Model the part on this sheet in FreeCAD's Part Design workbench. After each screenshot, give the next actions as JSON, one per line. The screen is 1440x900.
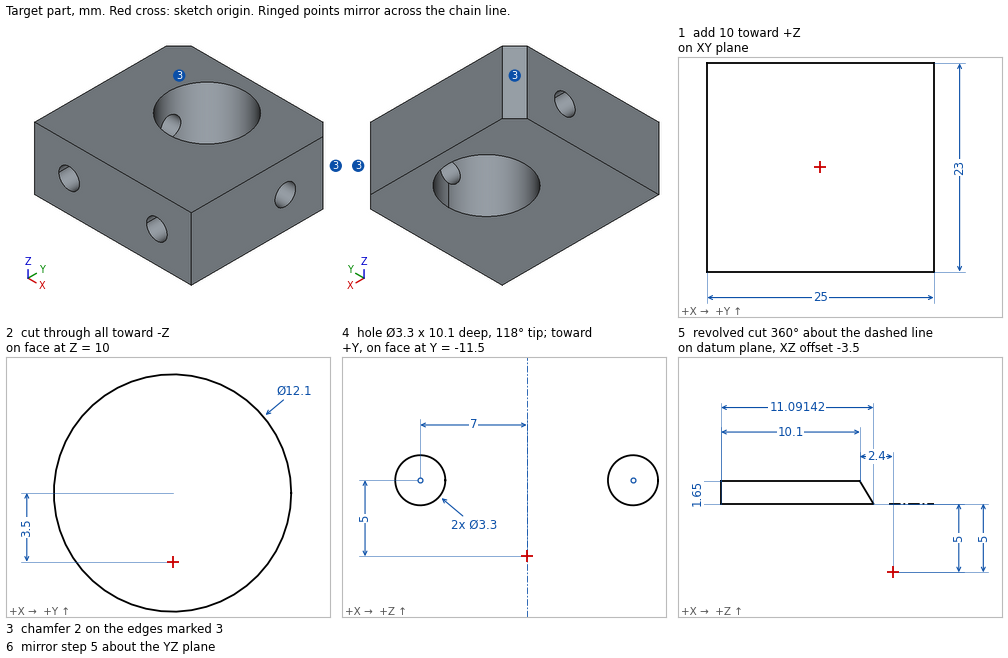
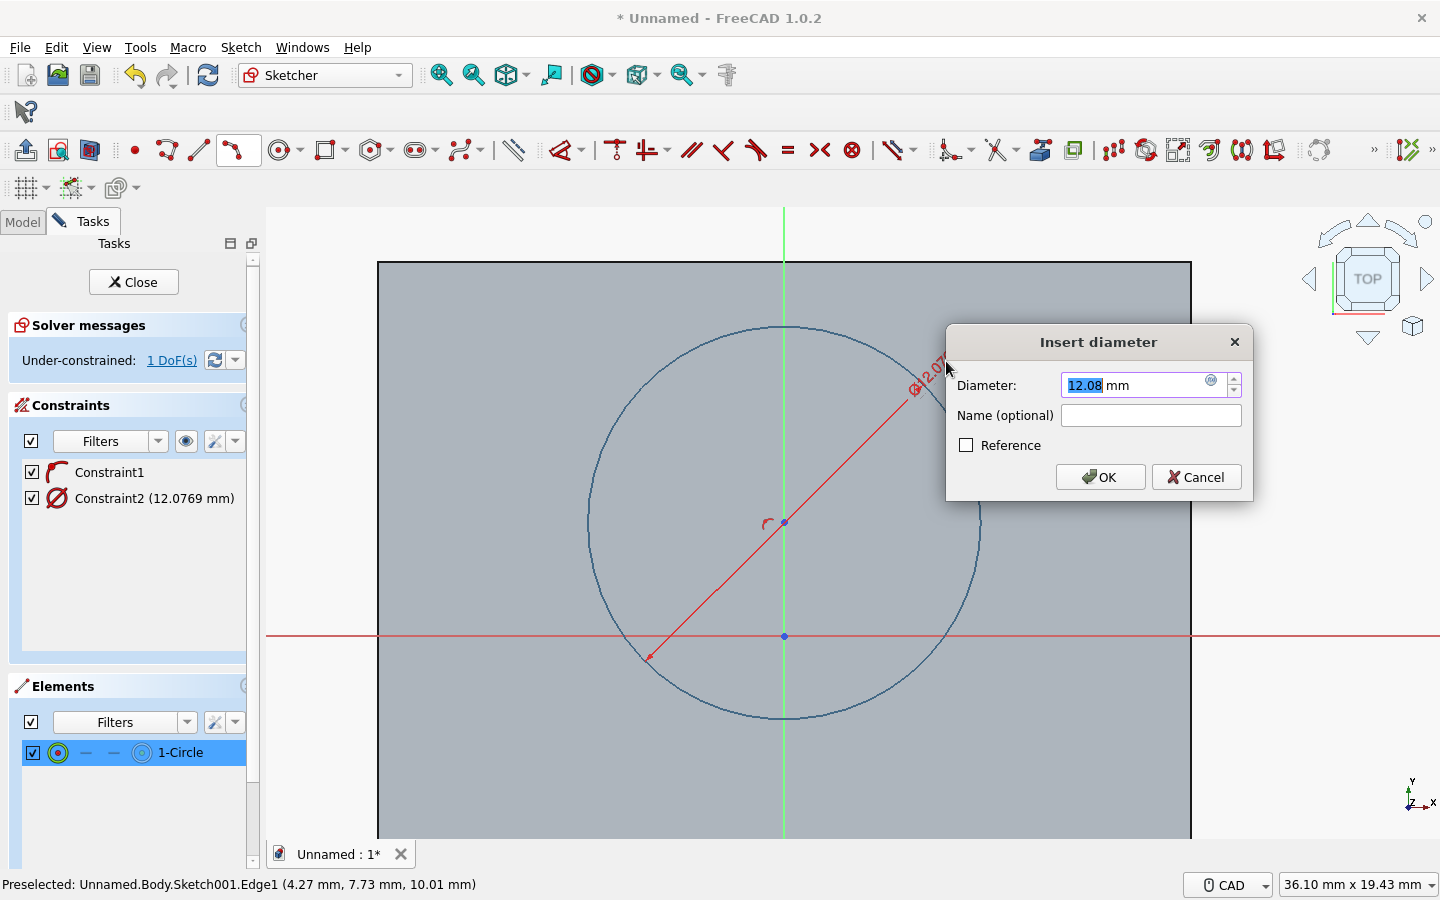
{"action": "type", "text": "12.1"}
{"action": "key", "text": "Return"}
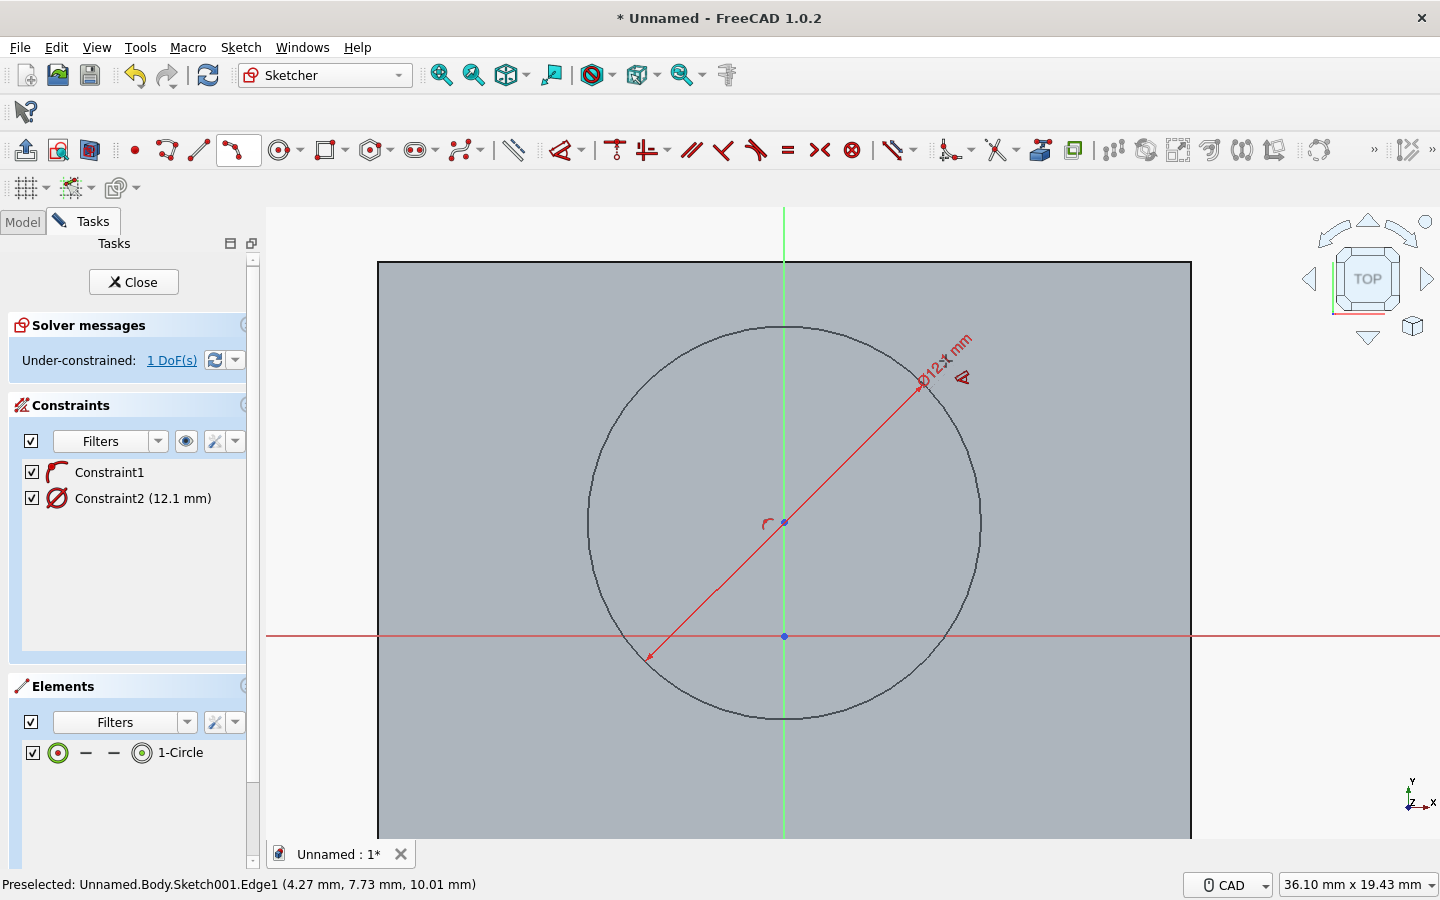
{"action": "left_click", "coordinate": [784, 523]}
{"action": "left_click", "coordinate": [818, 580]}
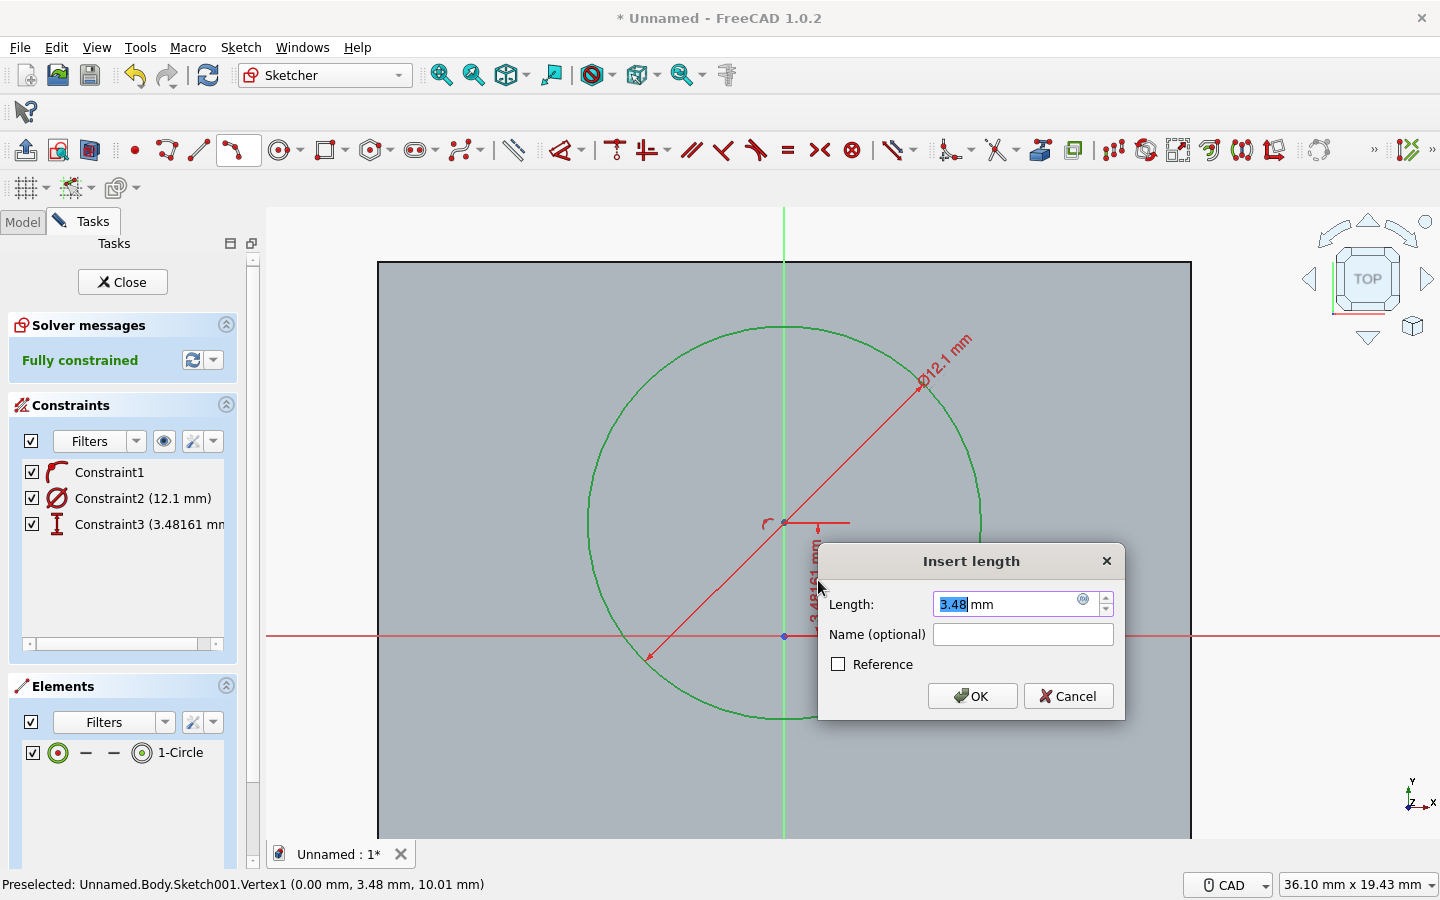
{"action": "type", "text": "3.5"}
{"action": "key", "text": "Return"}
{"action": "key", "text": "Escape"}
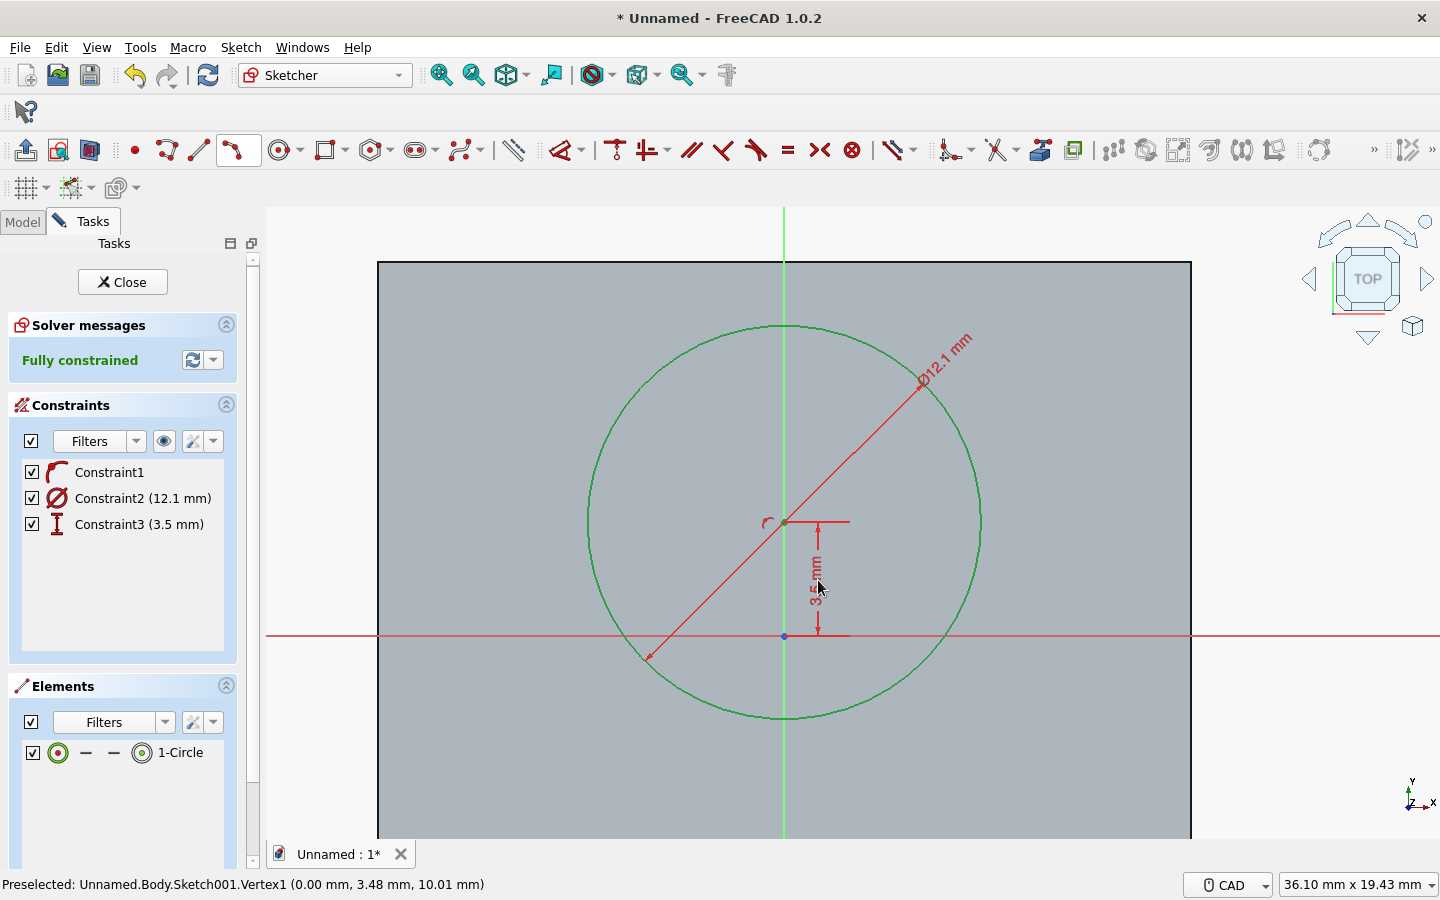
{"action": "left_click", "coordinate": [123, 282]}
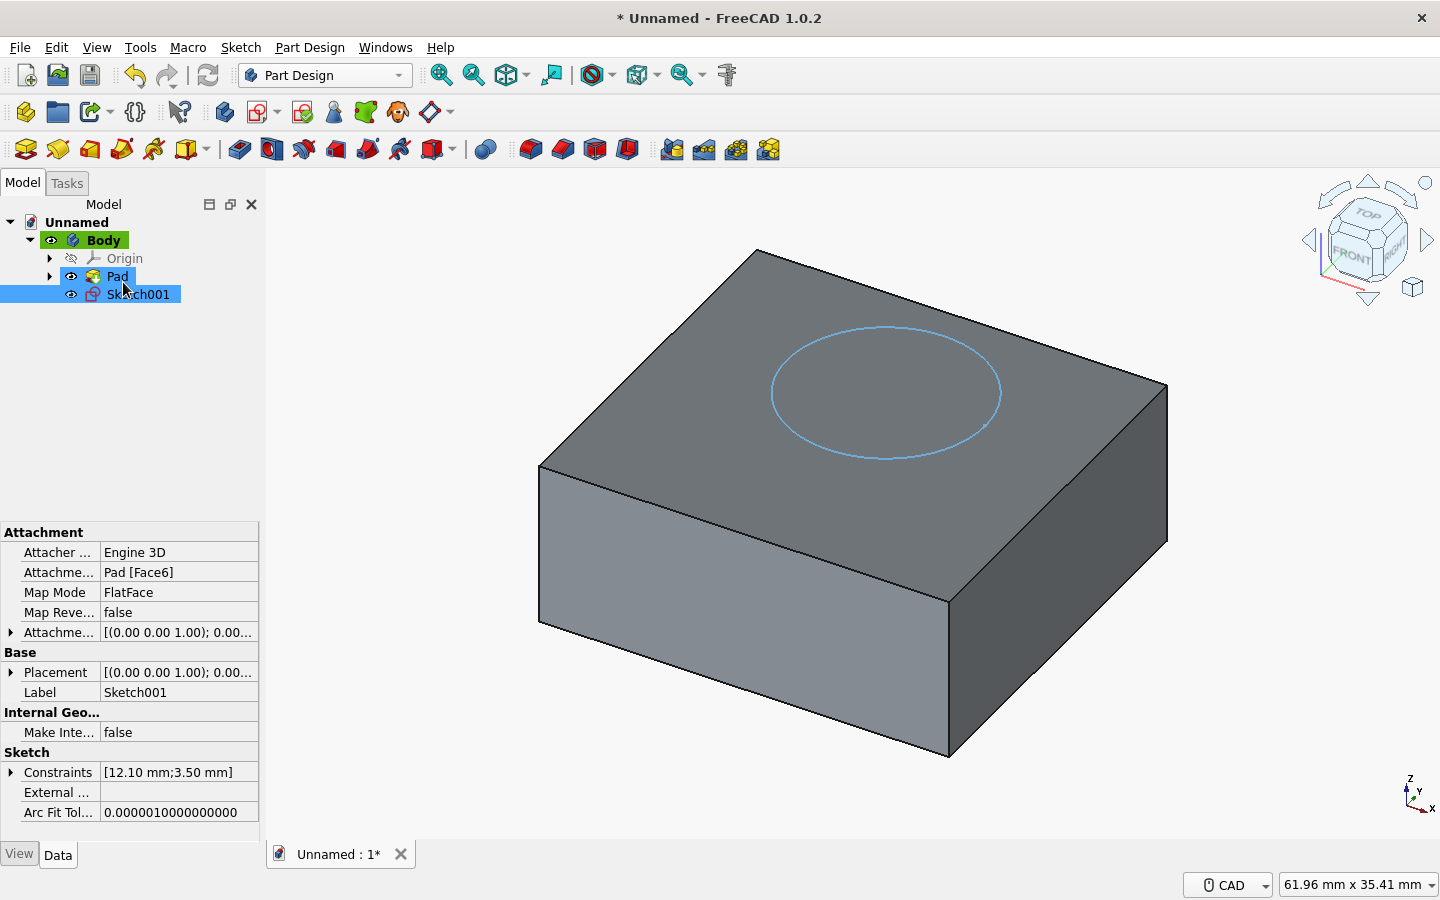
{"action": "left_click", "coordinate": [240, 150]}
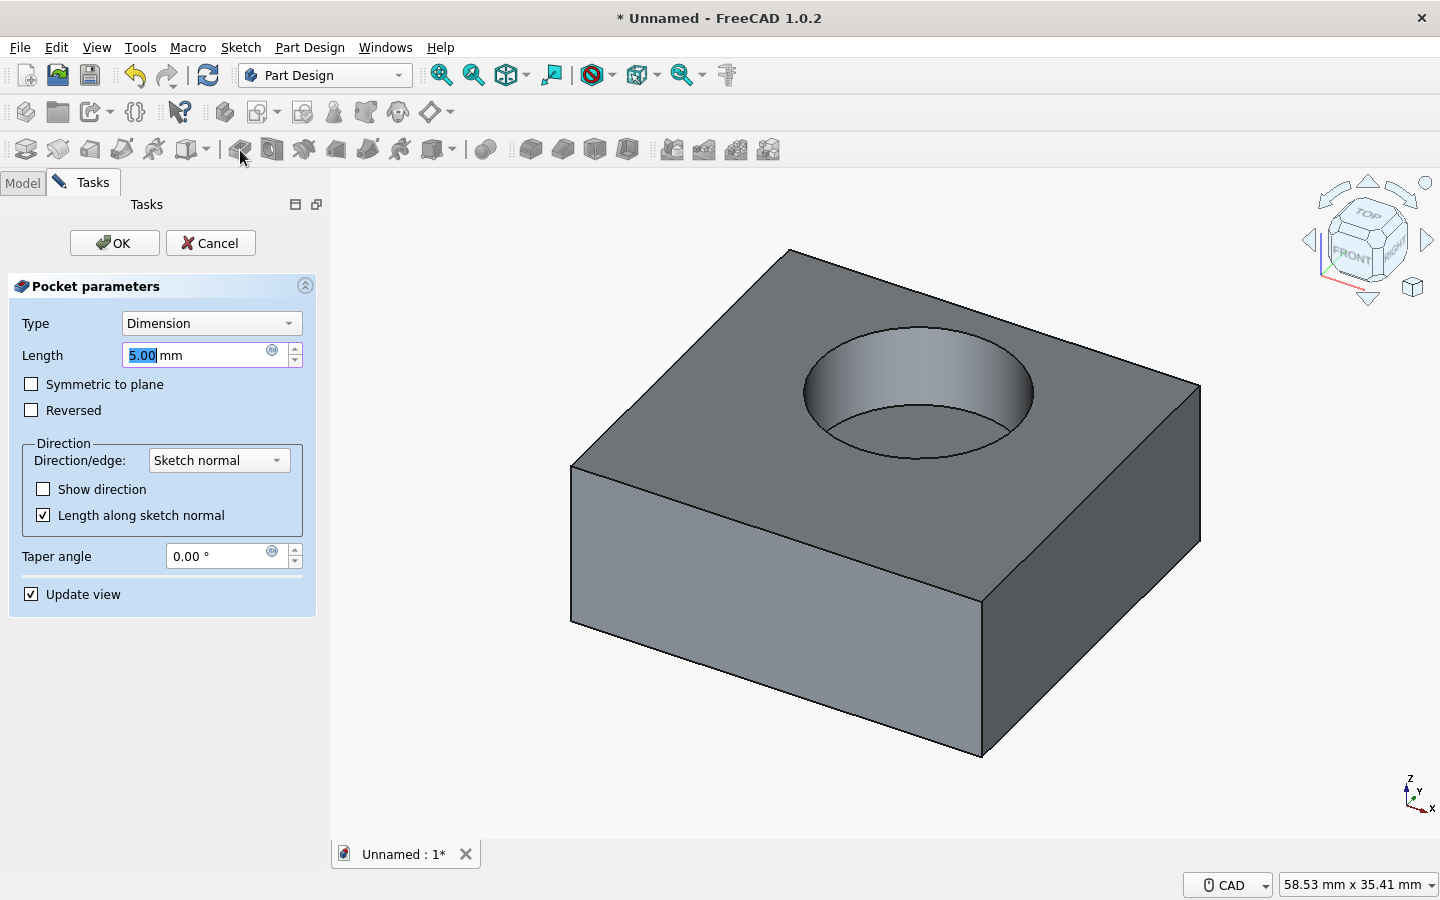
{"action": "left_click", "coordinate": [212, 324]}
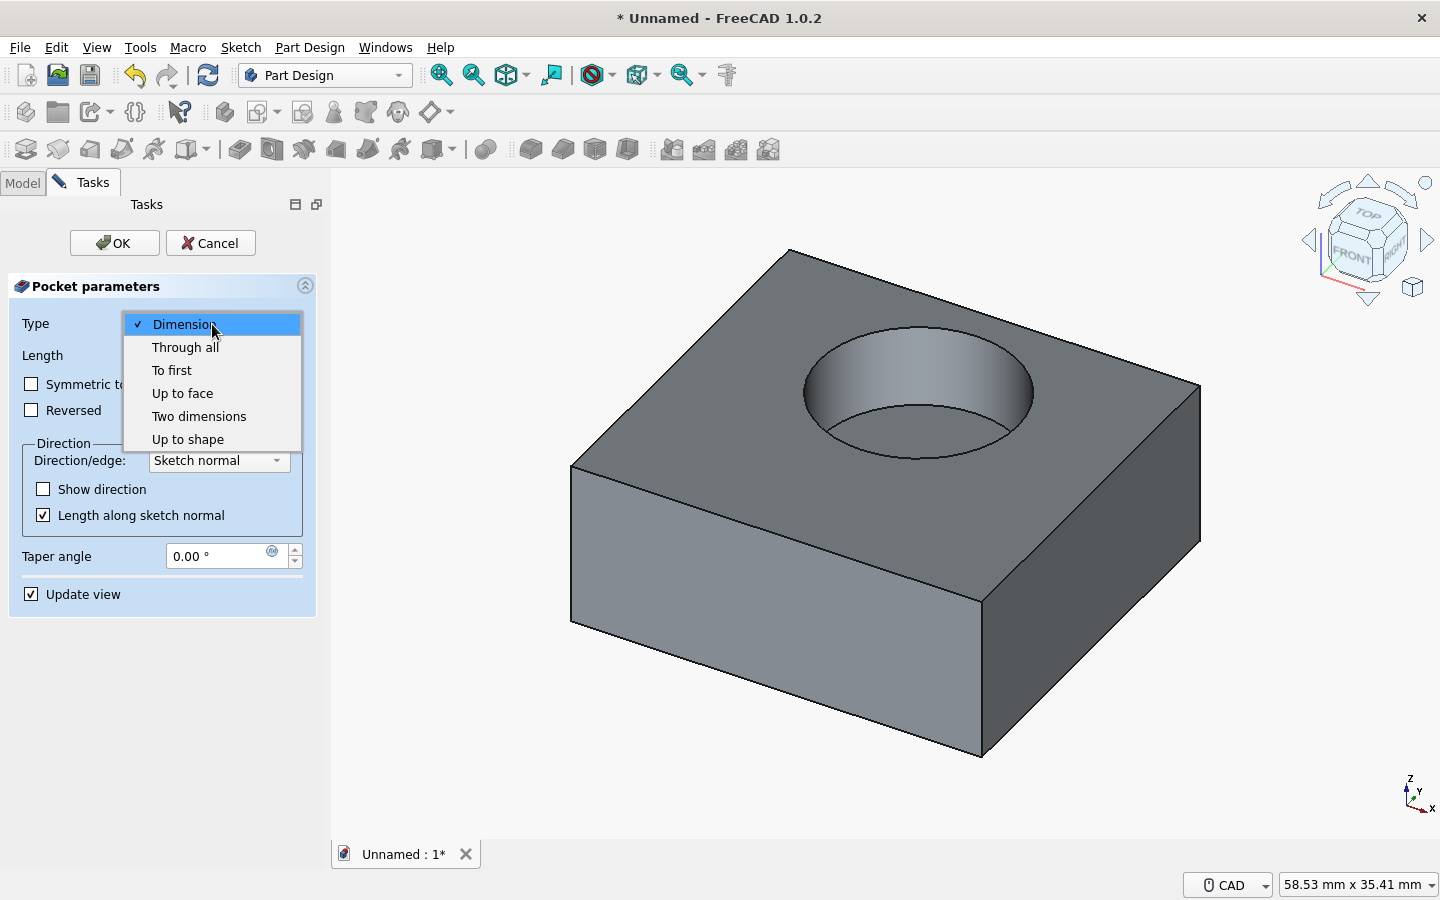
{"action": "left_click", "coordinate": [212, 348]}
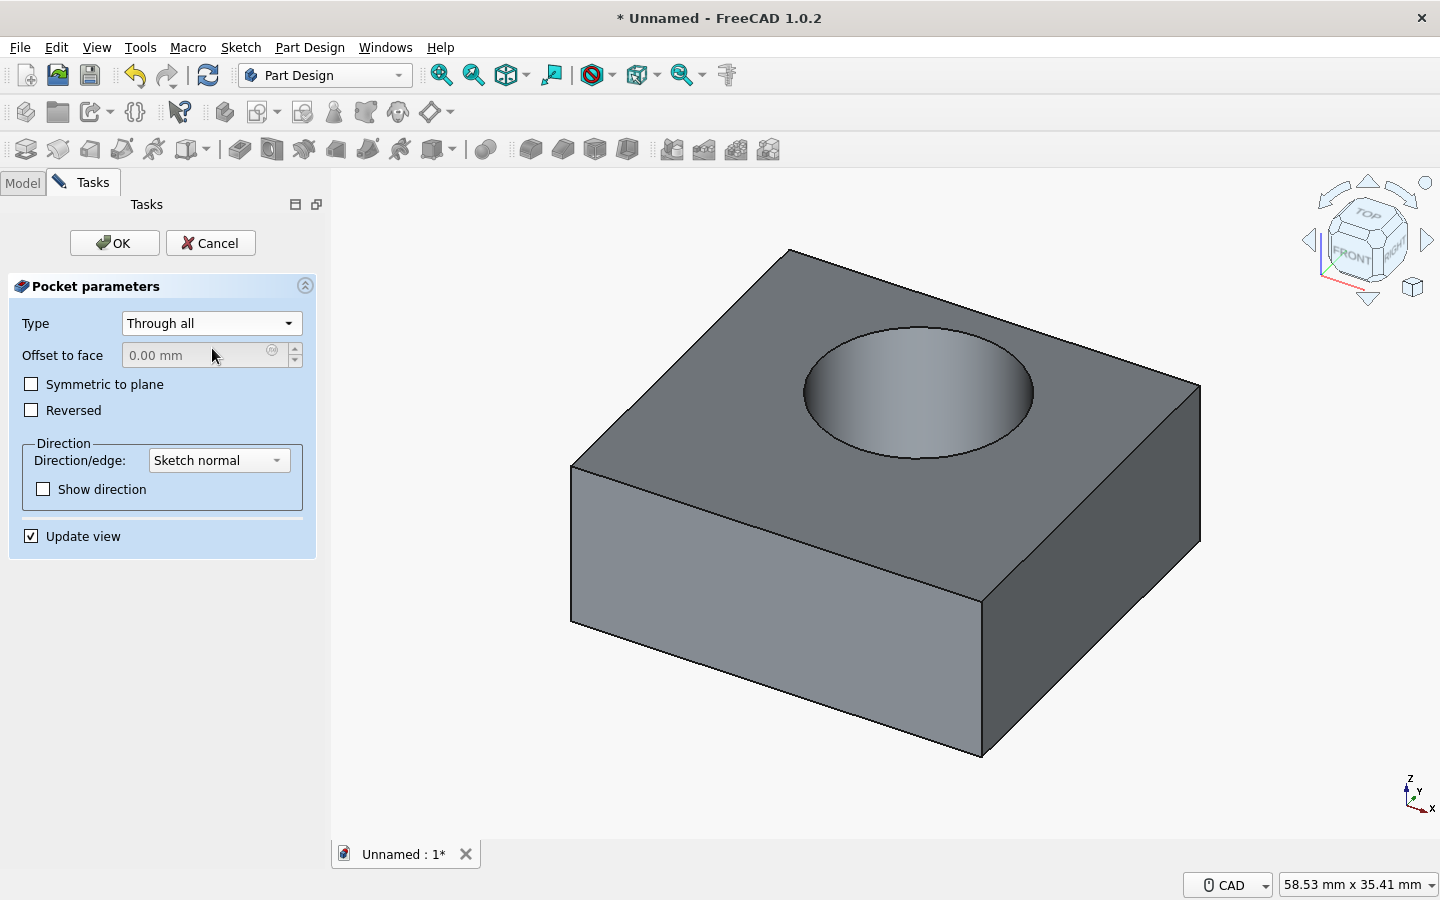
{"action": "left_click", "coordinate": [115, 243]}